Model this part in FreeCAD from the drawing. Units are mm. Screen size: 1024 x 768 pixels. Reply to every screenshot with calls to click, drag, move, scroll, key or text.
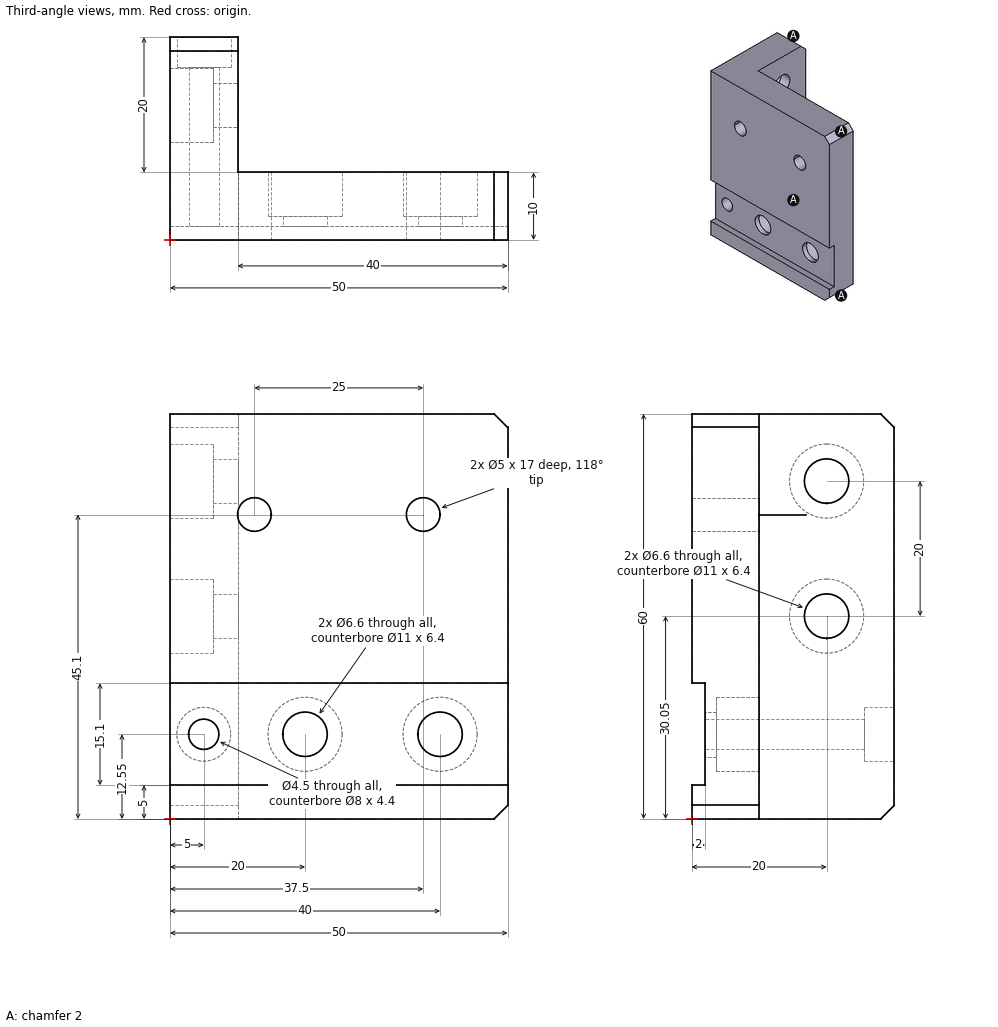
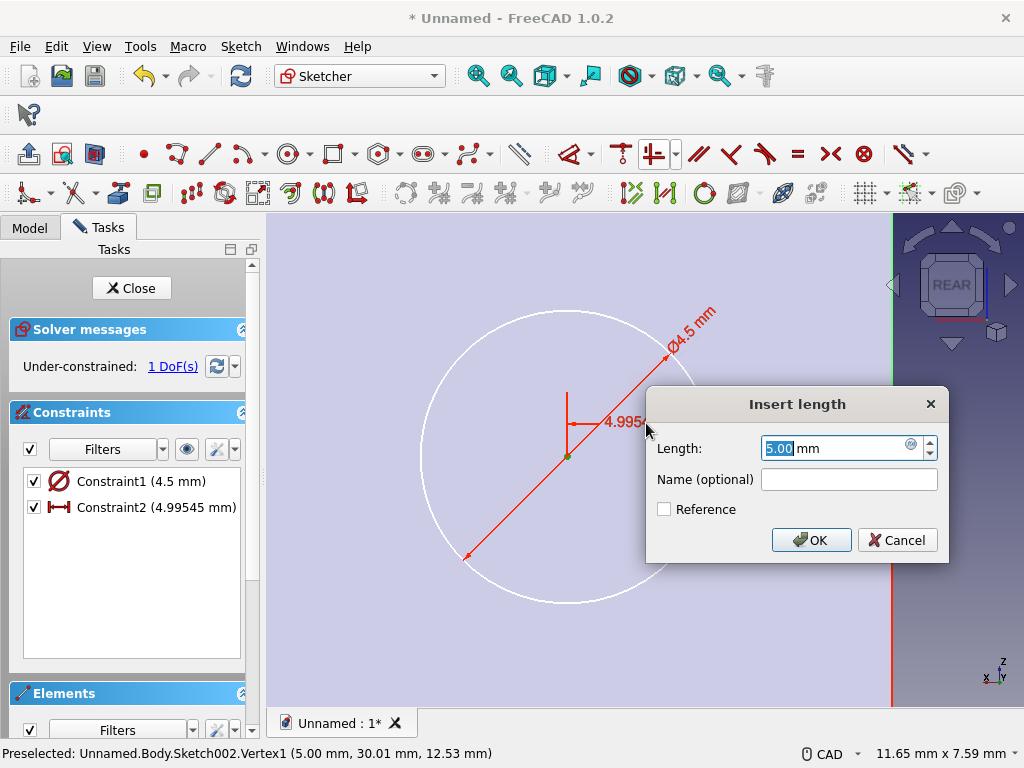
text(5)
key(Return)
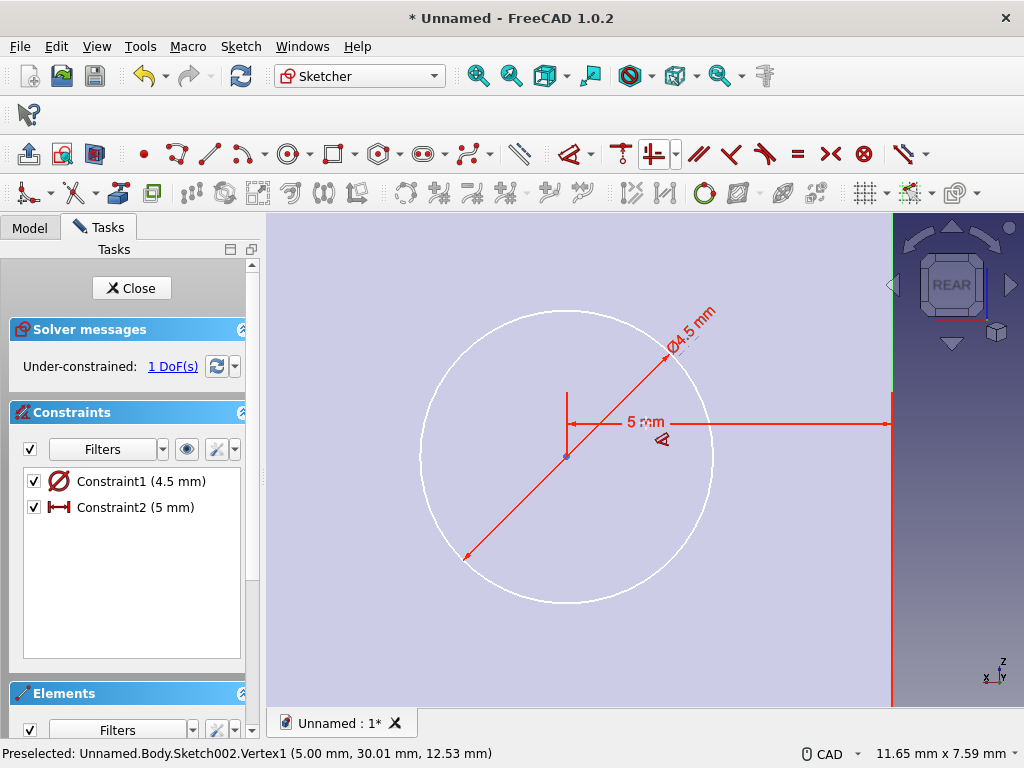
click(567, 457)
click(533, 568)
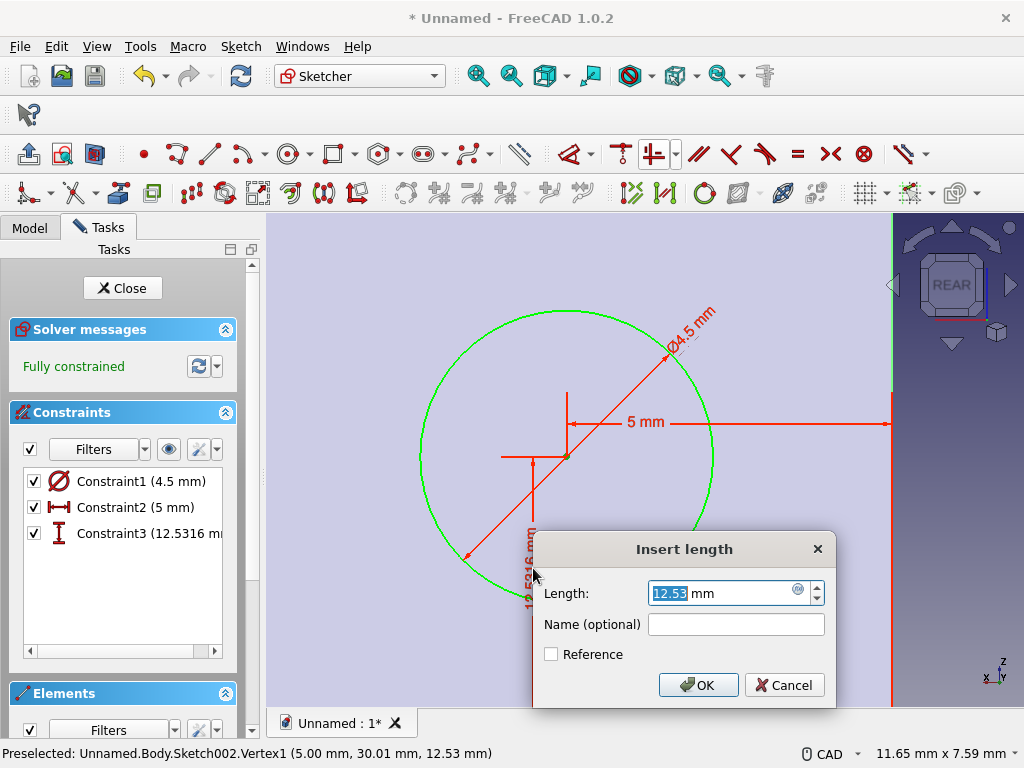
text(12.55)
key(Return)
key(Escape)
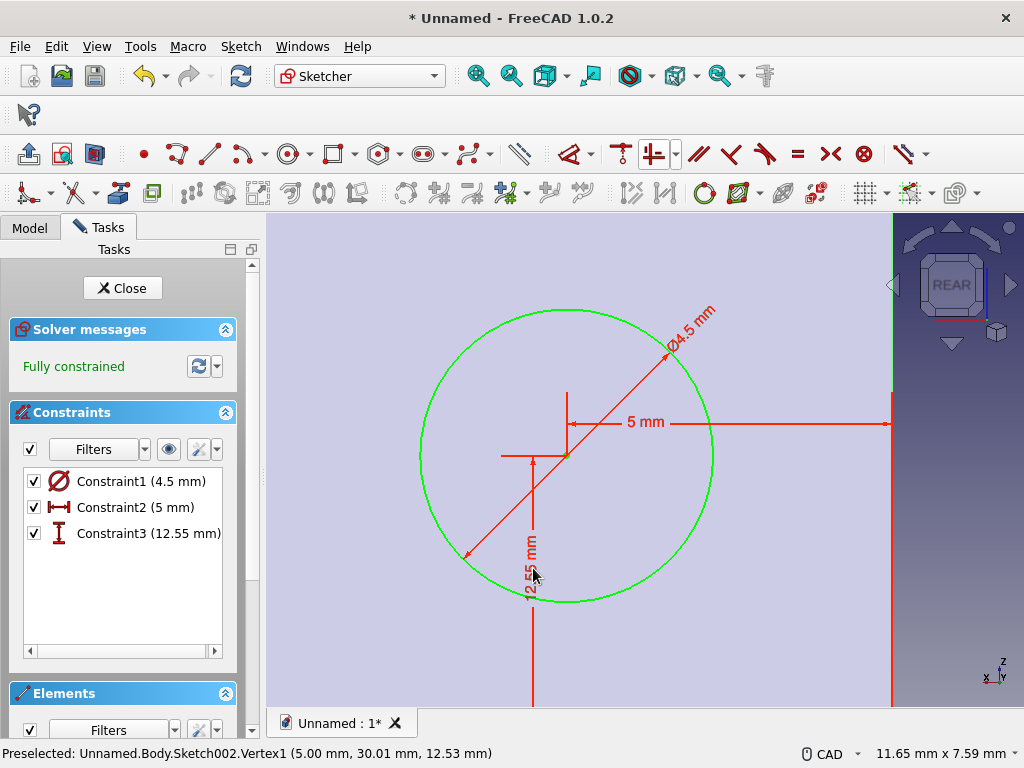
click(123, 288)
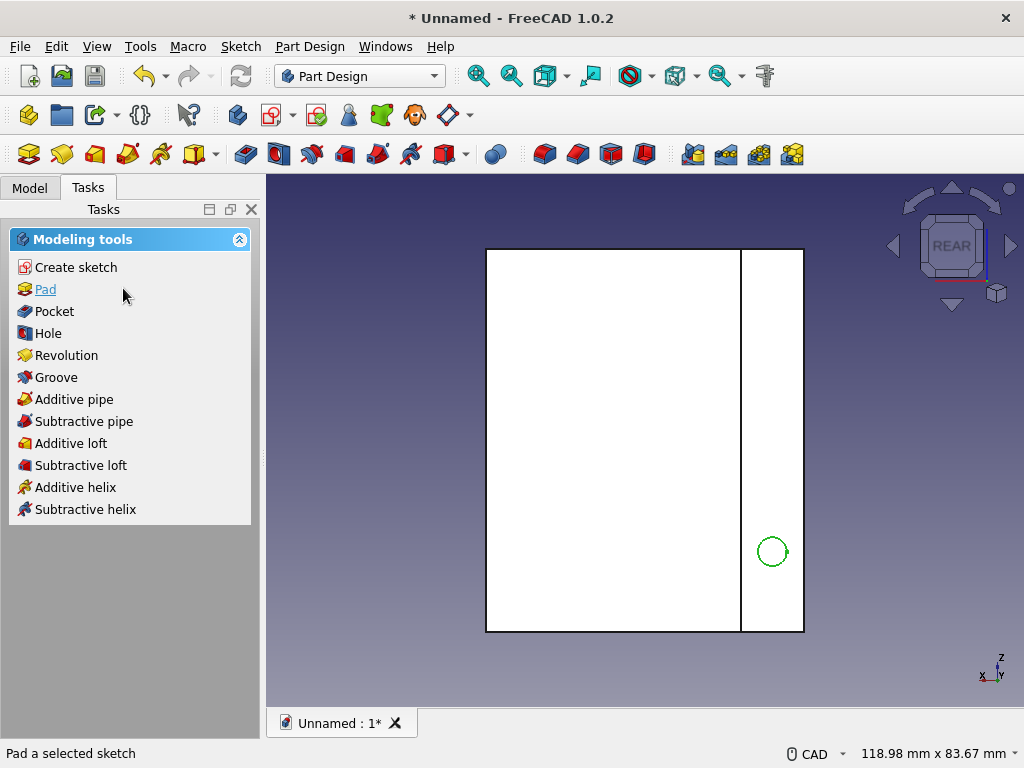
click(279, 154)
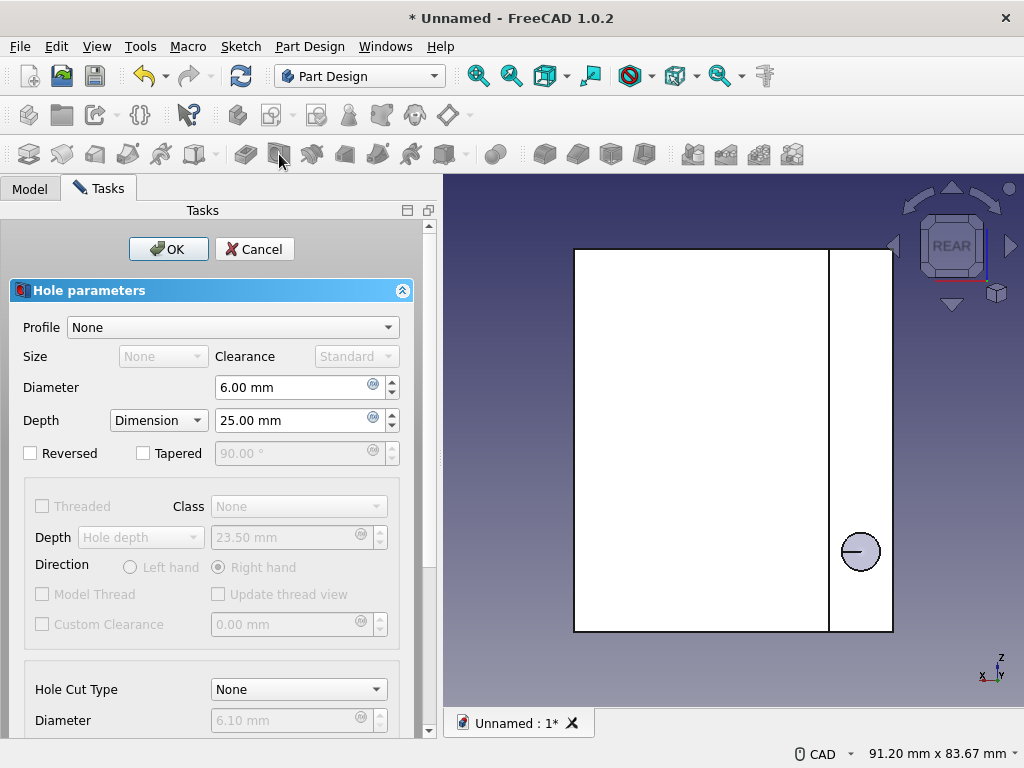
triple_click(300, 388)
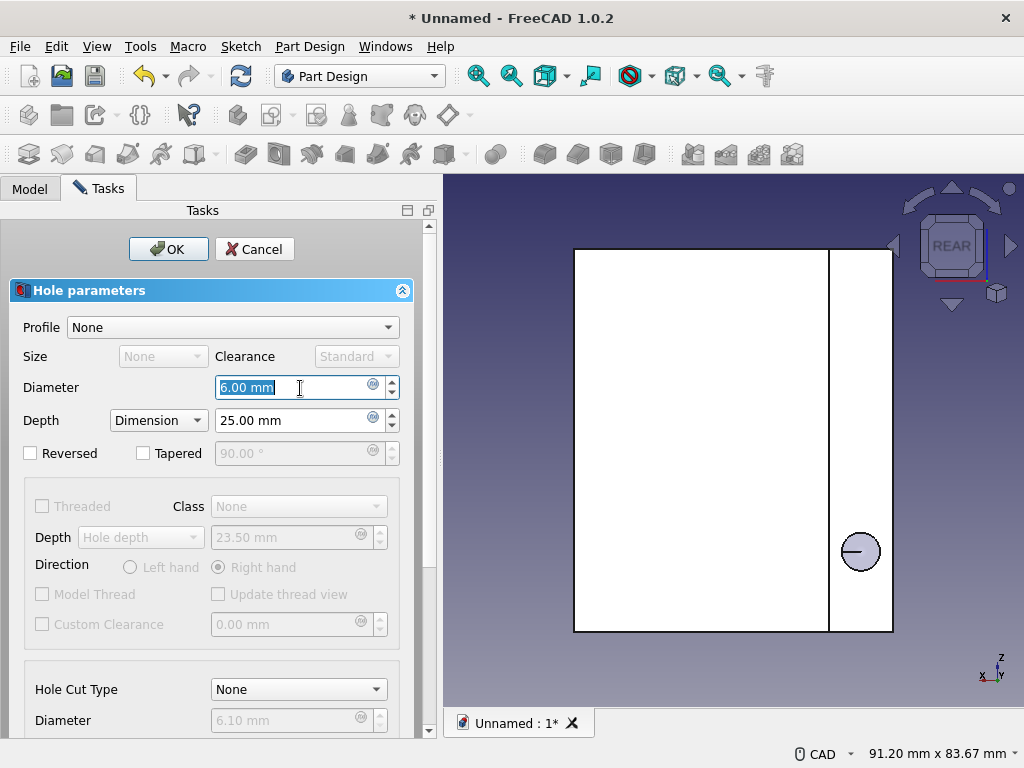
text(4.5)
key(Tab)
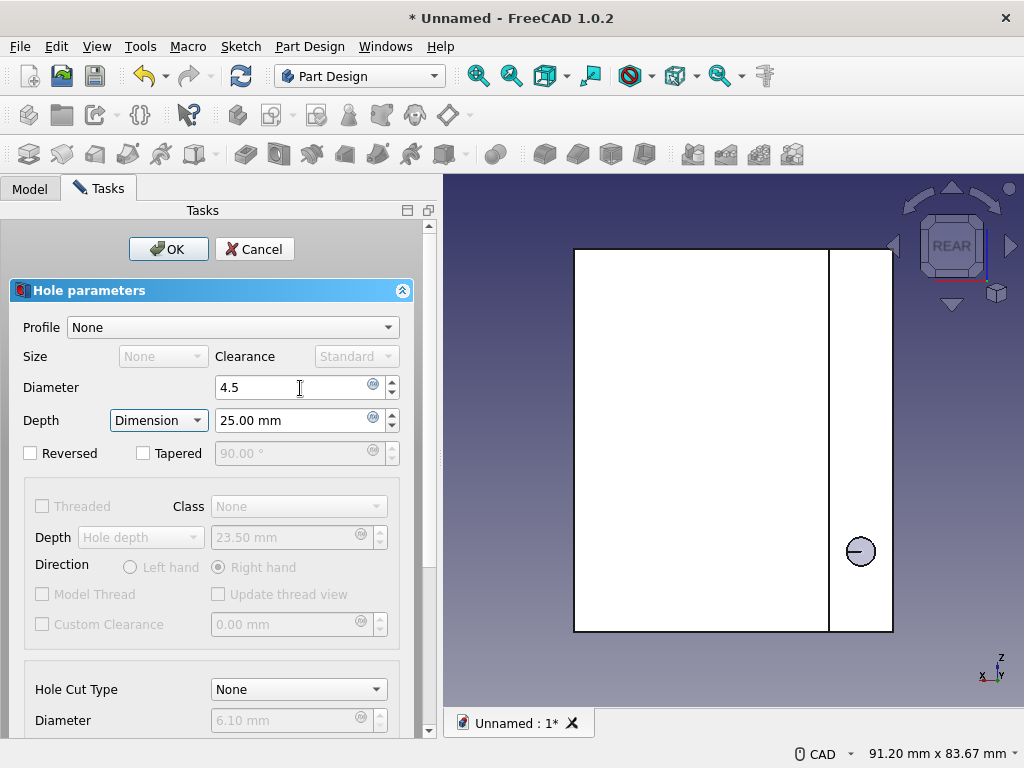
click(160, 420)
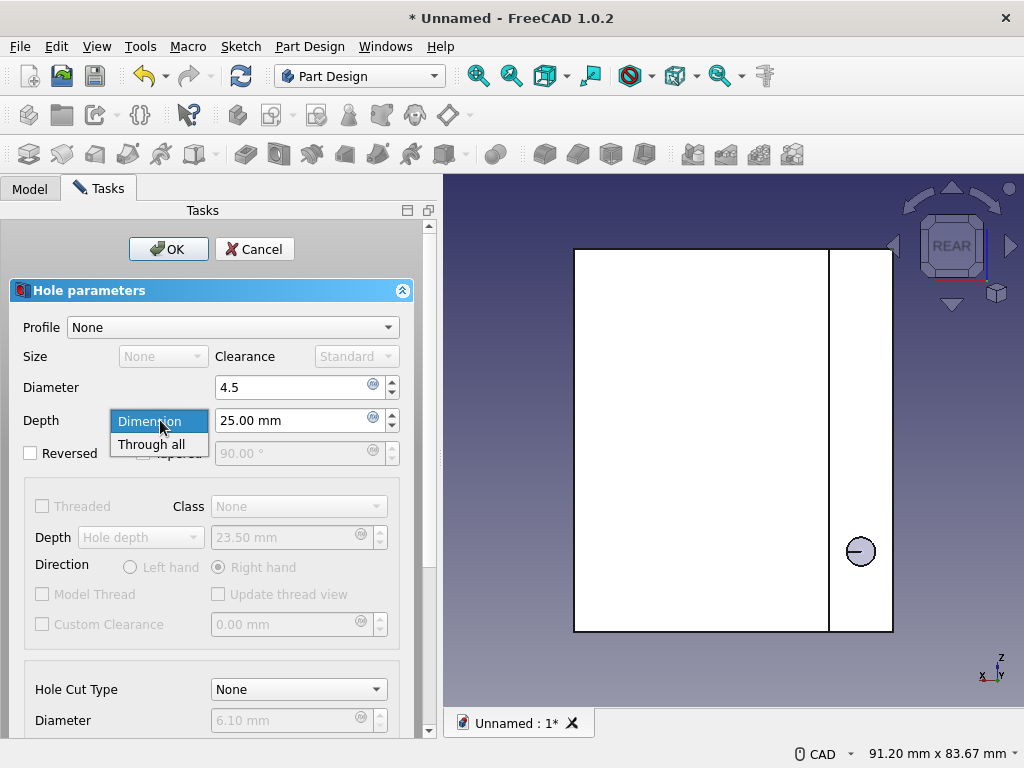
click(158, 444)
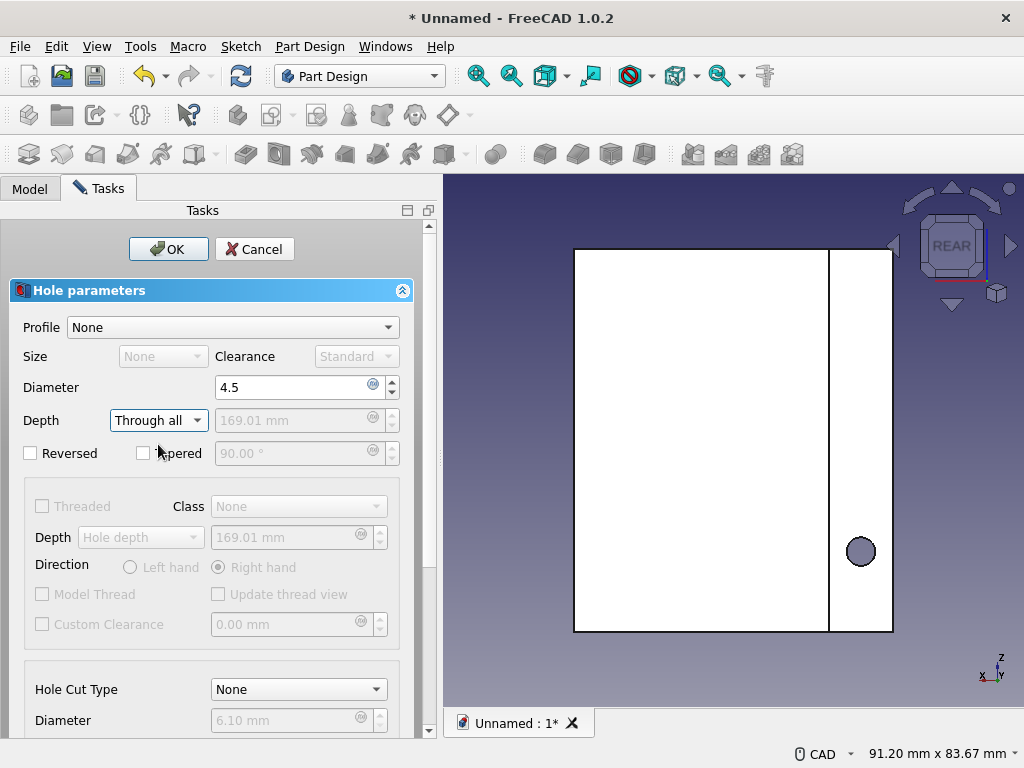
click(300, 690)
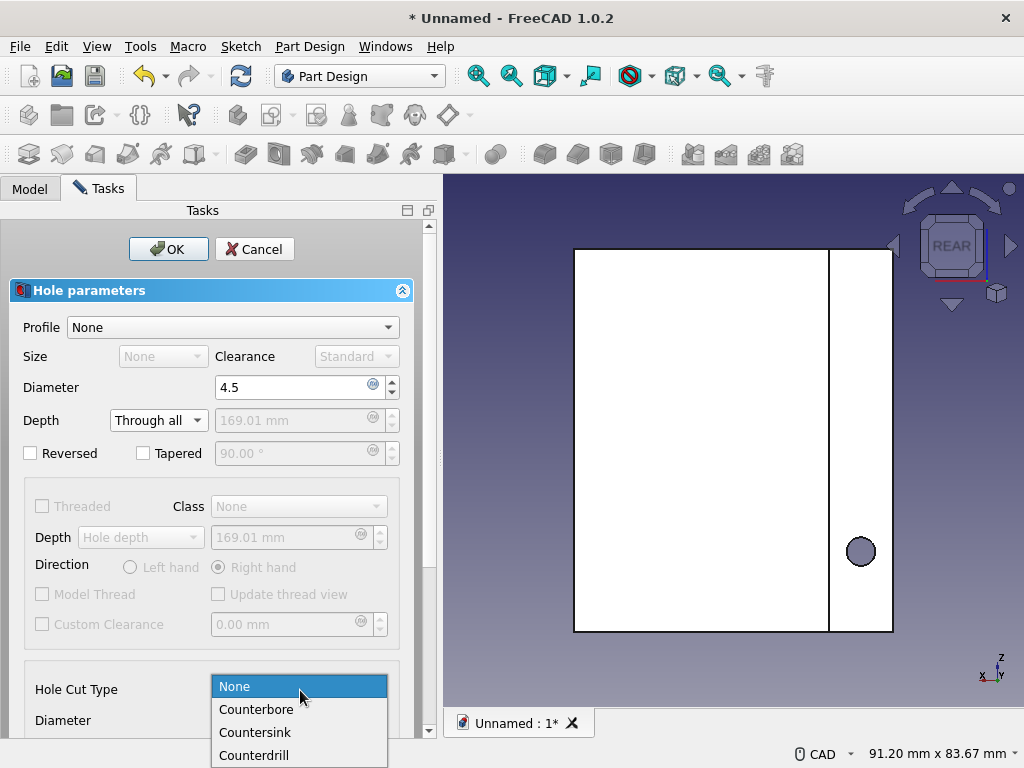
click(298, 710)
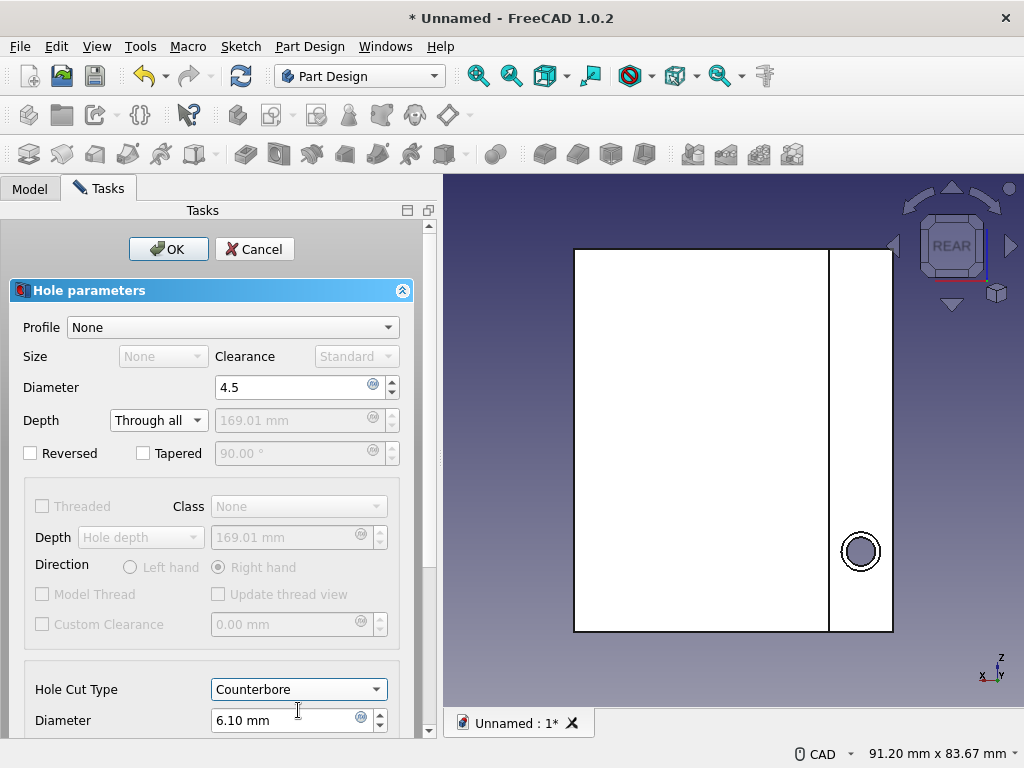
triple_click(292, 720)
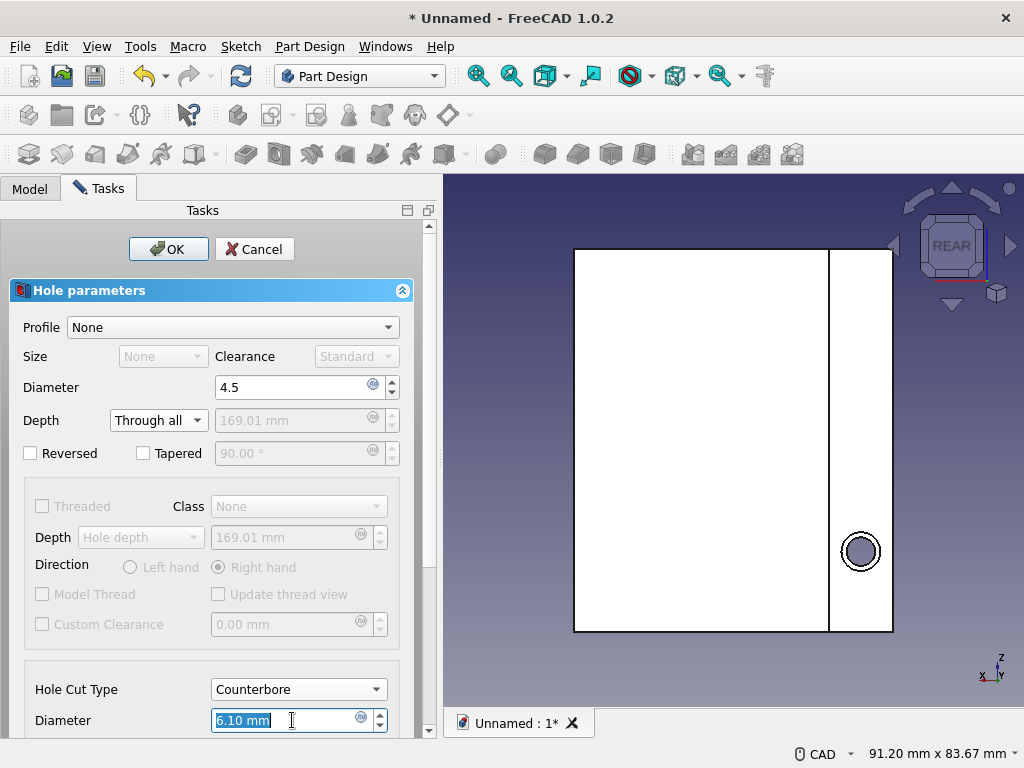
text(8)
key(Tab)